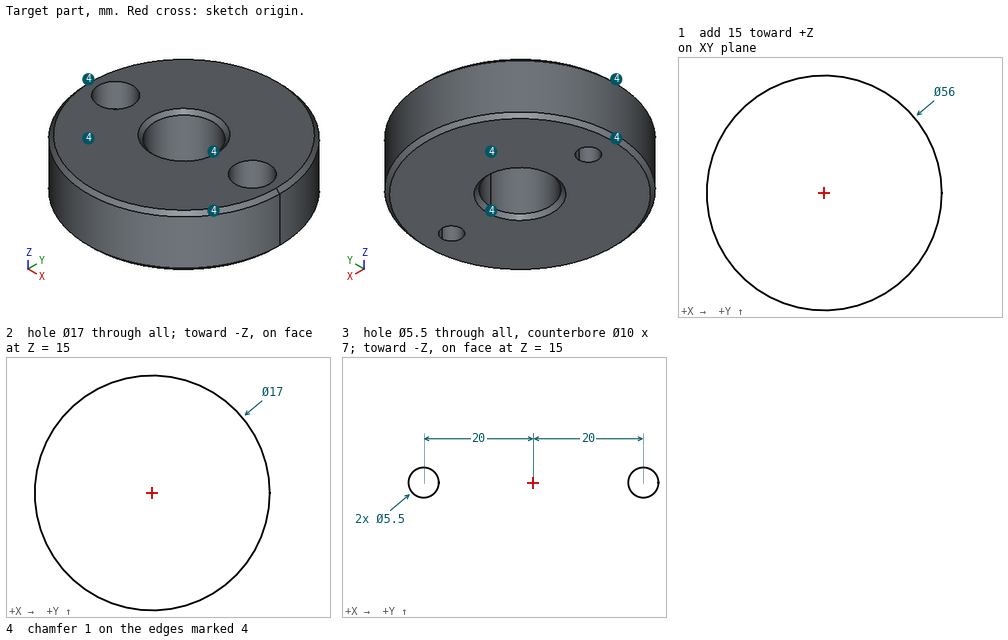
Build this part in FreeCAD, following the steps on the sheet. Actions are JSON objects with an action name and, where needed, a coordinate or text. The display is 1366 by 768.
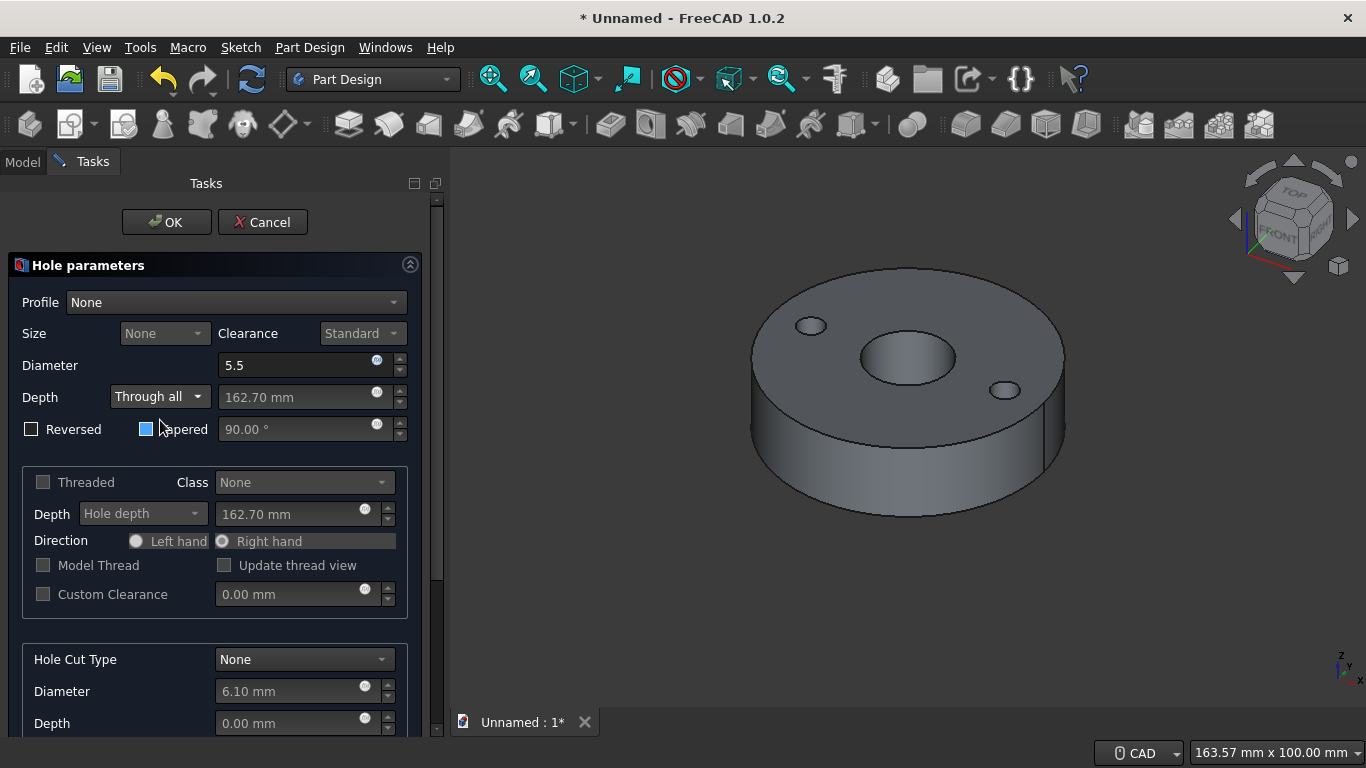
{"action": "left_click", "coordinate": [306, 660]}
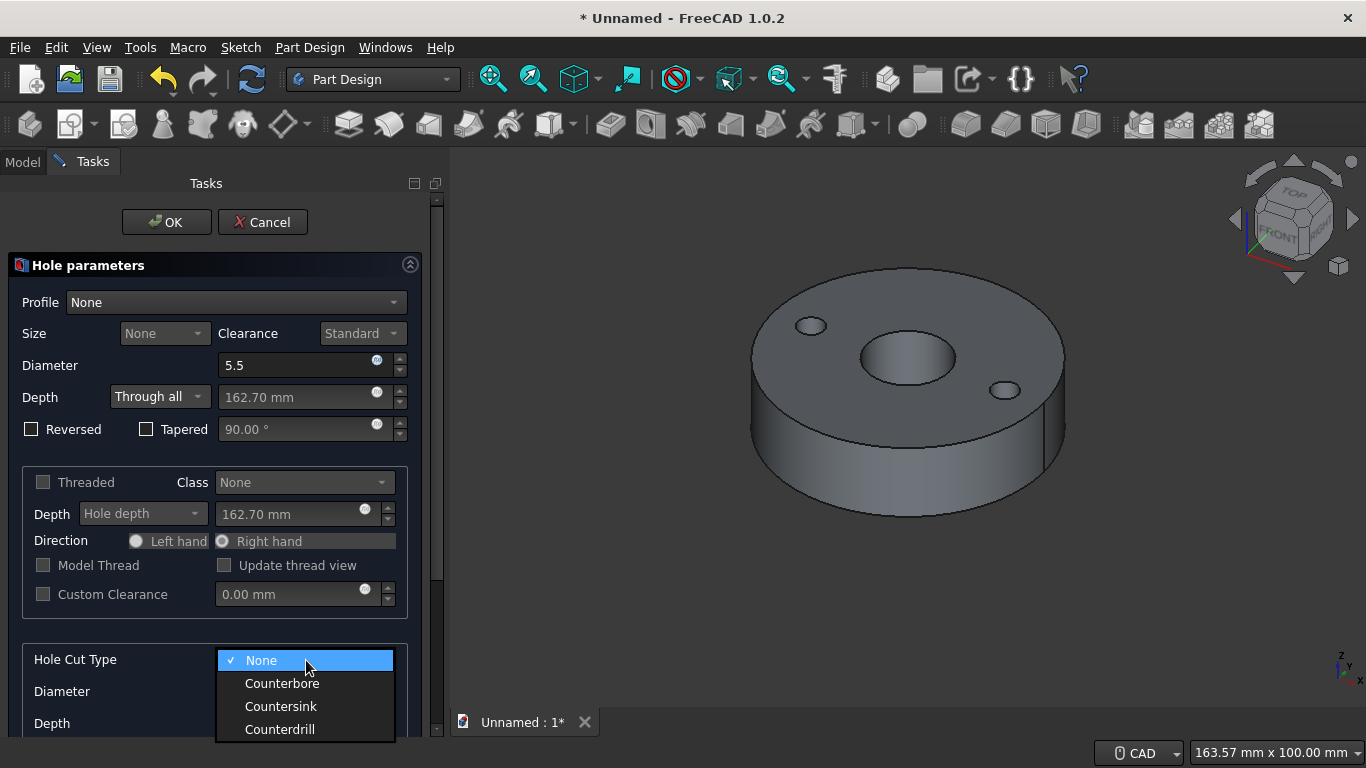
{"action": "left_click", "coordinate": [304, 684]}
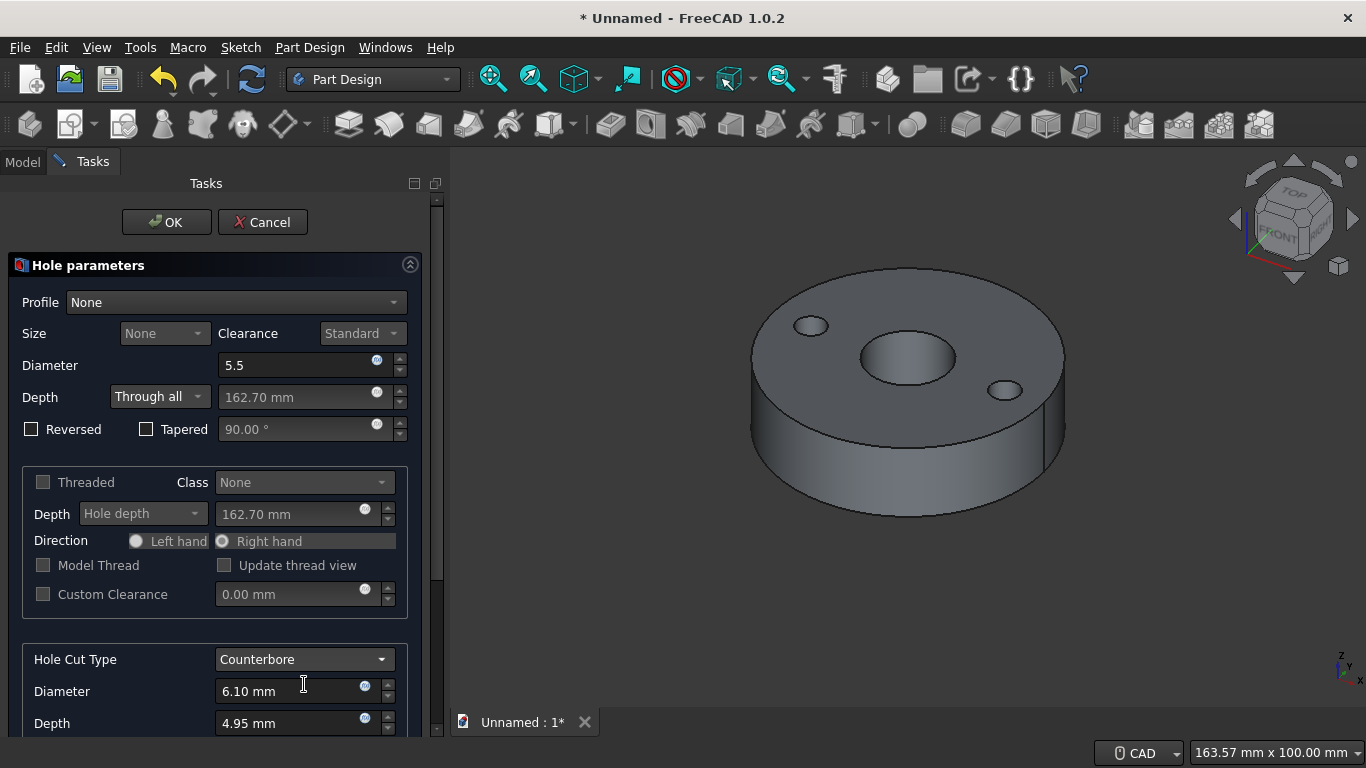
{"action": "triple_click", "coordinate": [298, 691]}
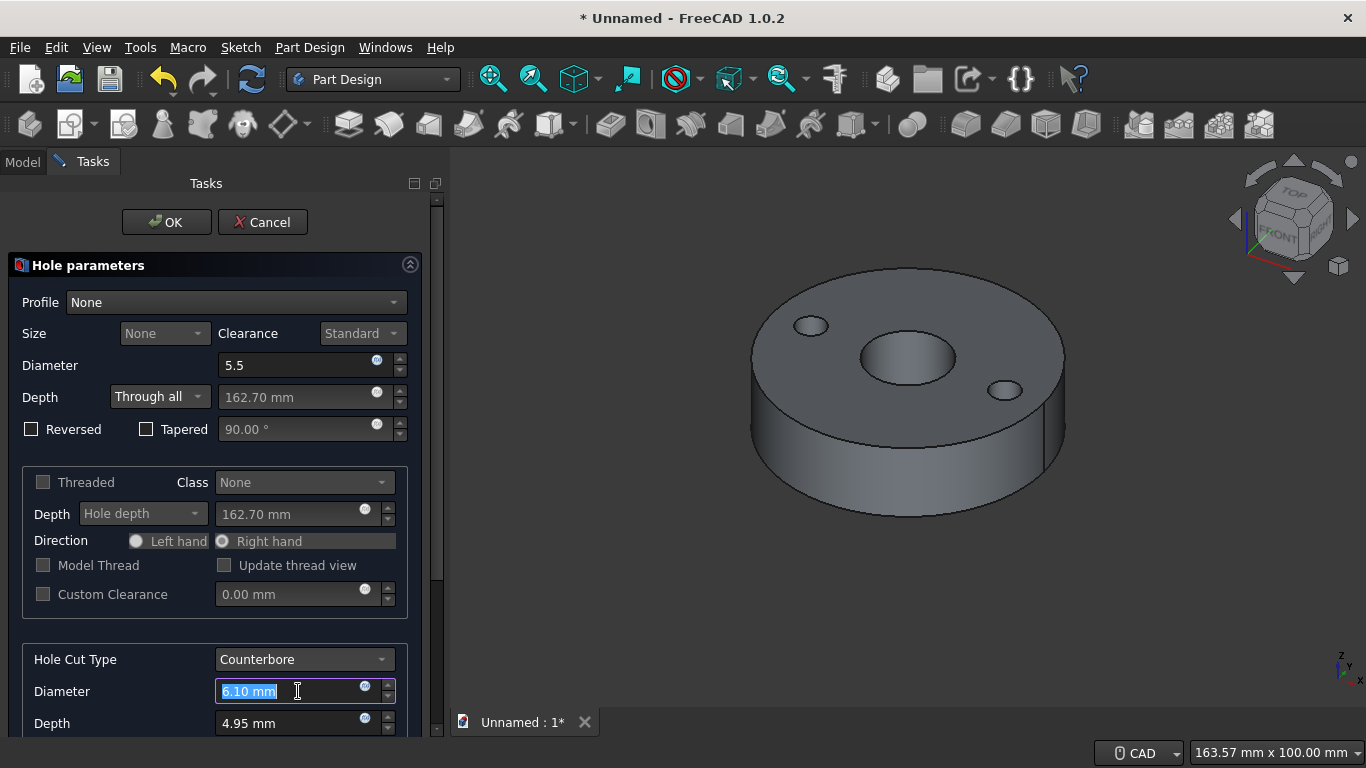
{"action": "type", "text": "10"}
{"action": "key", "text": "Tab"}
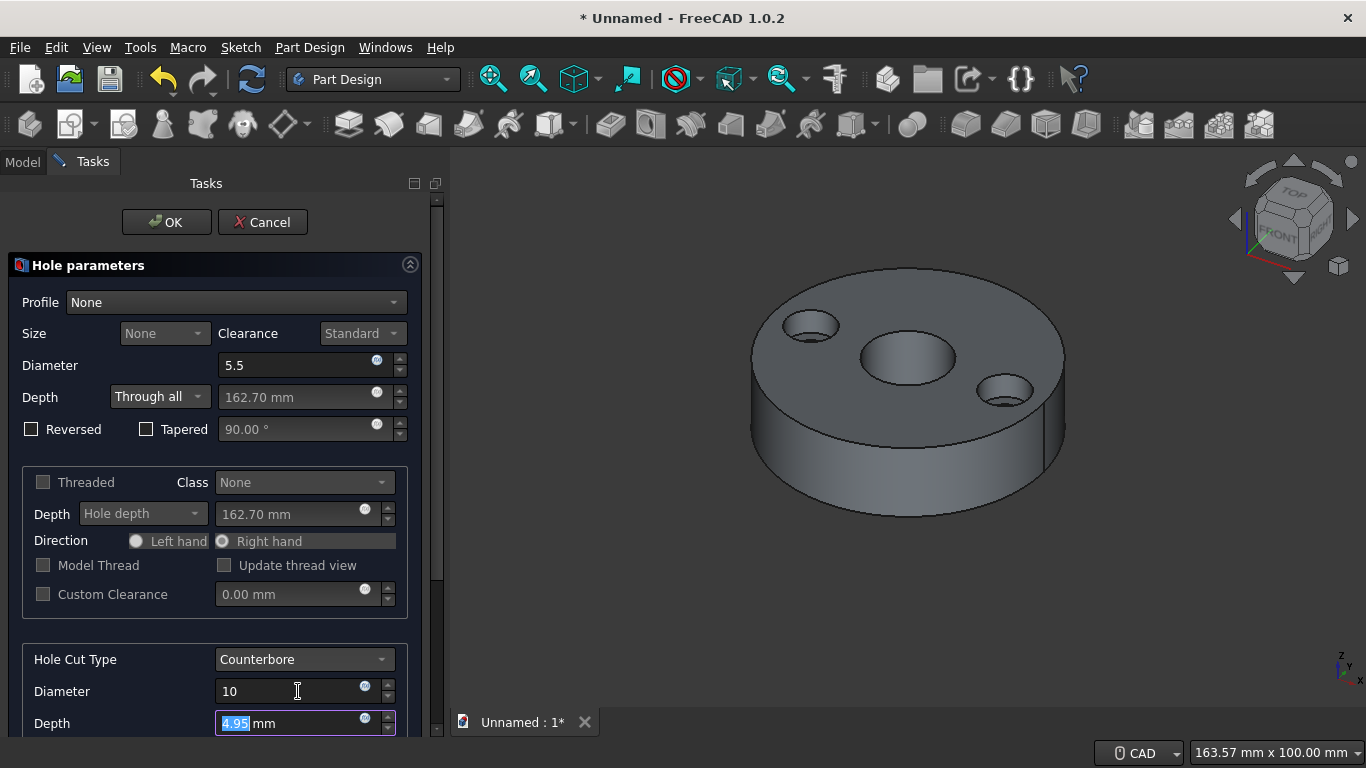
{"action": "type", "text": "7"}
{"action": "key", "text": "Tab"}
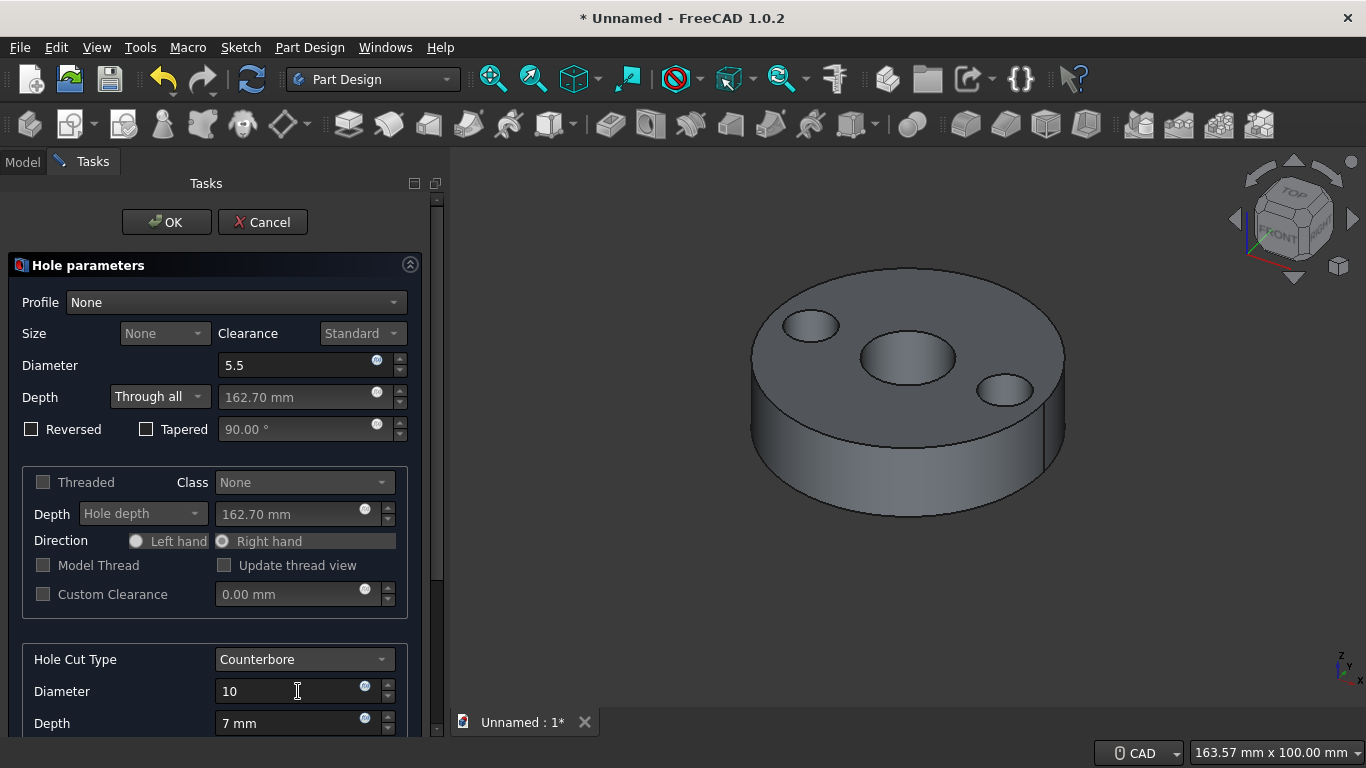
{"action": "left_click", "coordinate": [167, 222]}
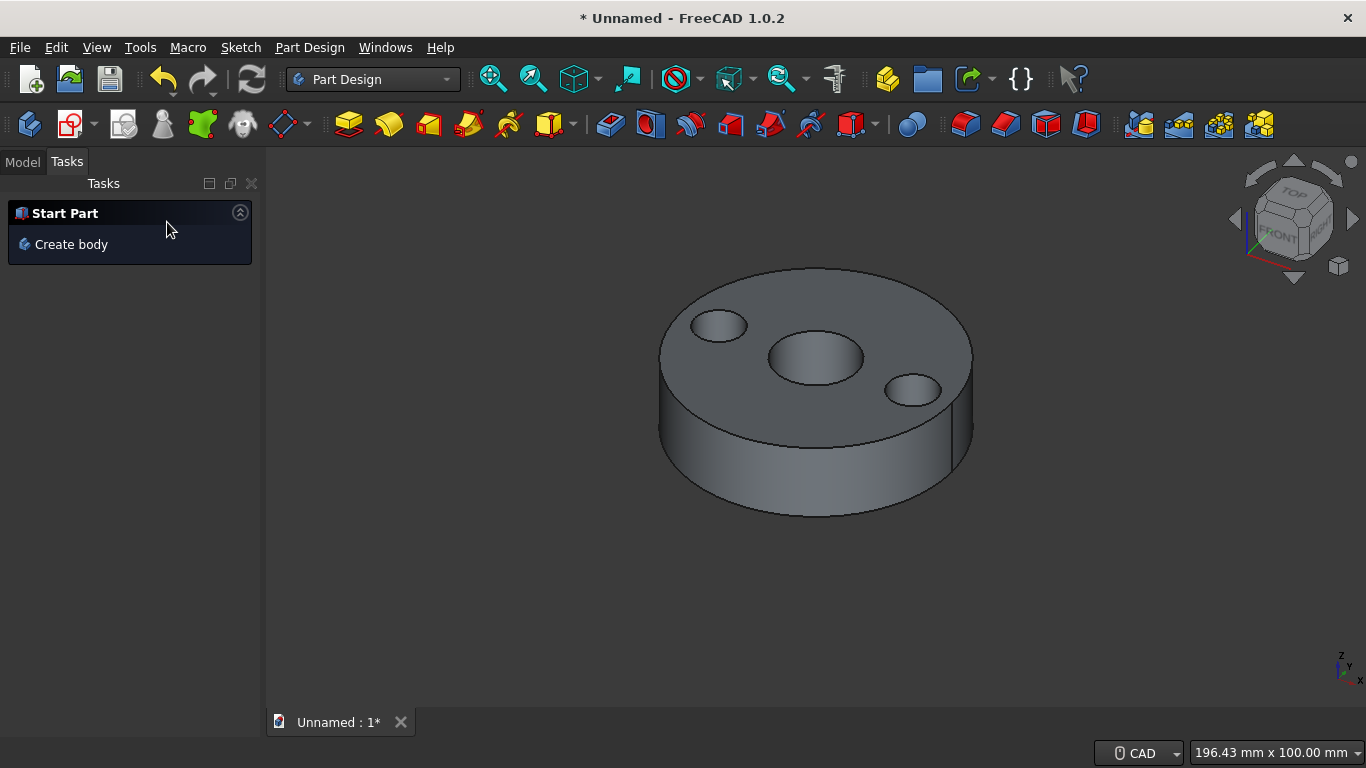
{"action": "left_click", "coordinate": [660, 367]}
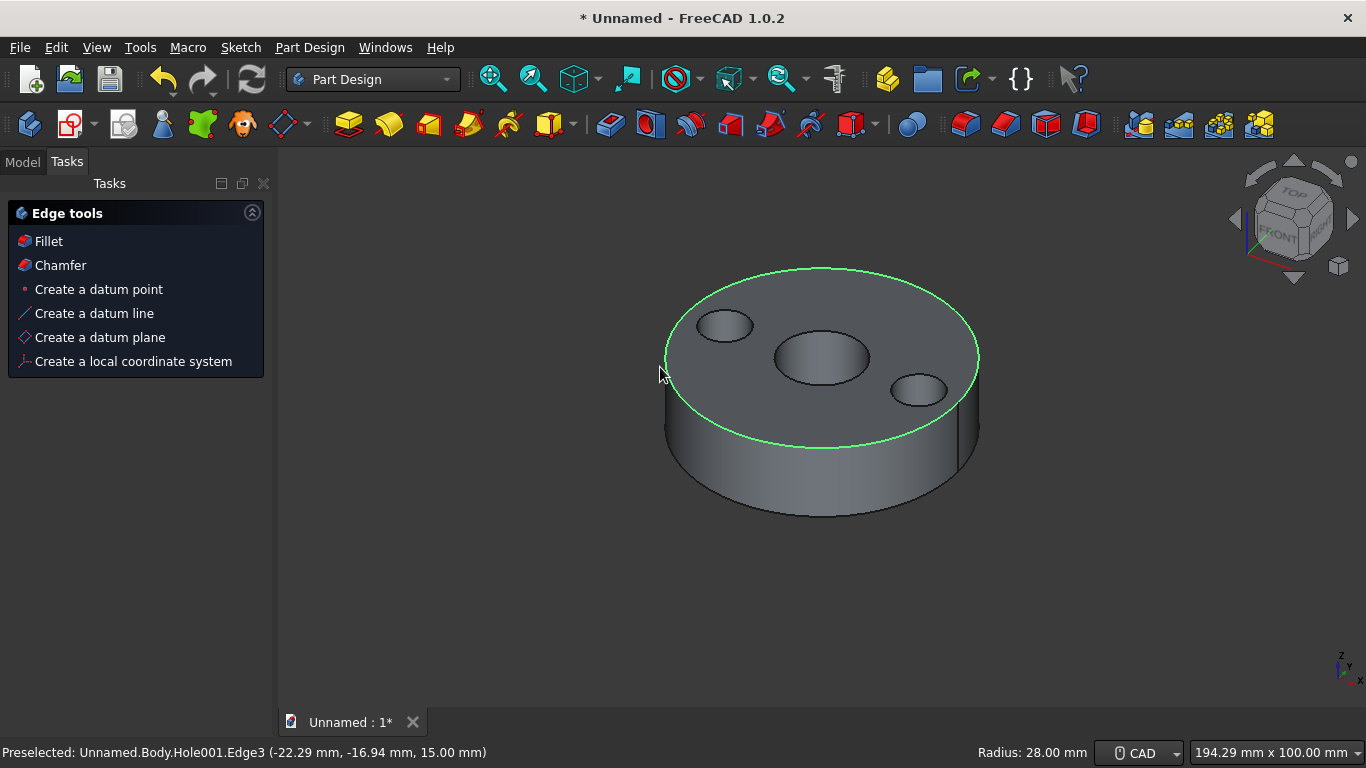
{"action": "left_click", "coordinate": [781, 344], "text": "ctrl"}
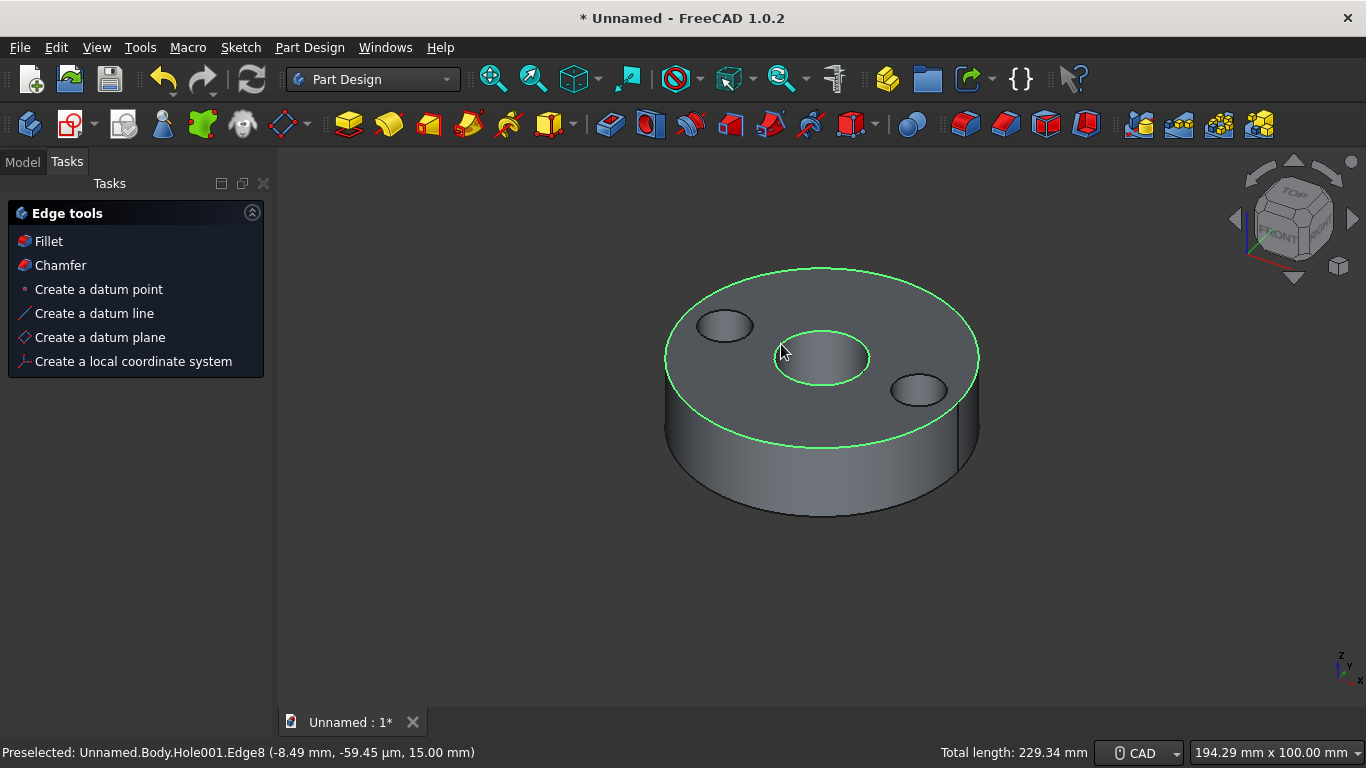
{"action": "key", "text": "0"}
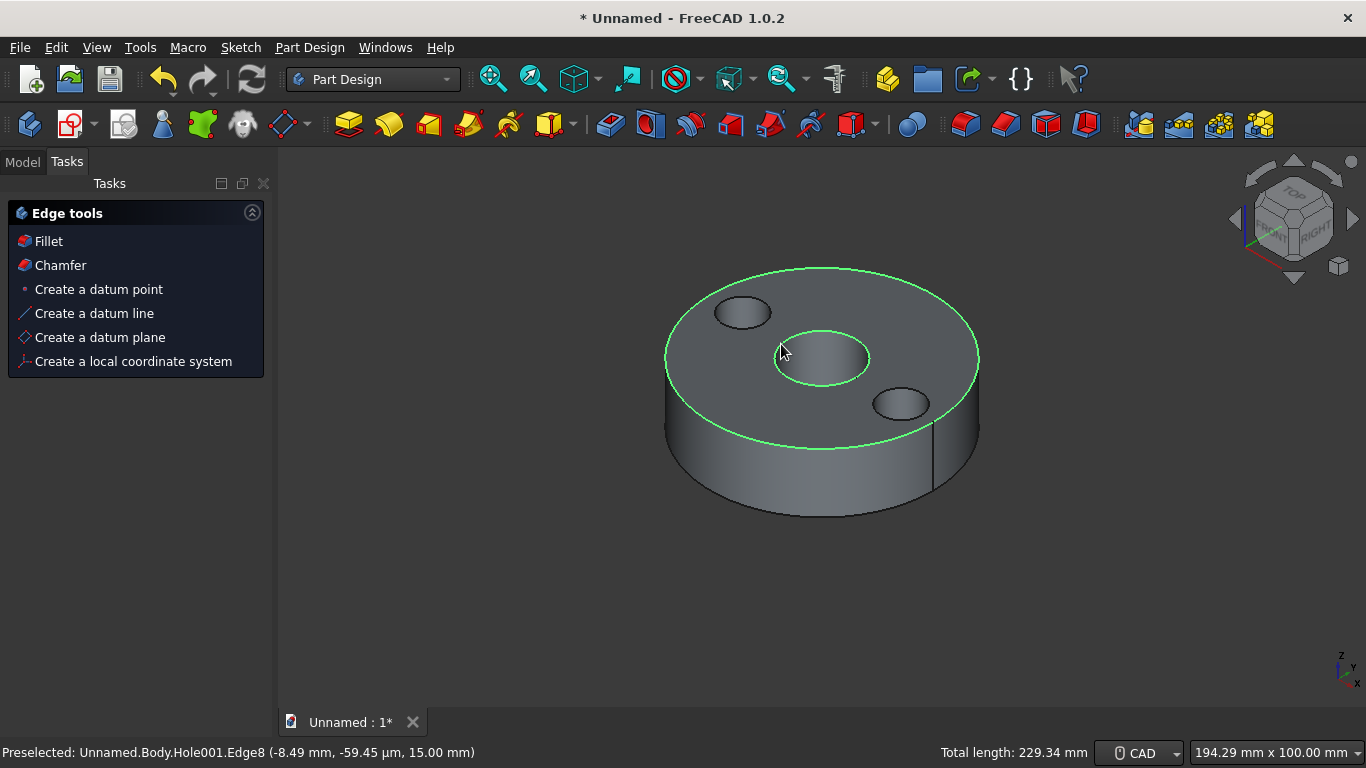
{"action": "key", "text": "2"}